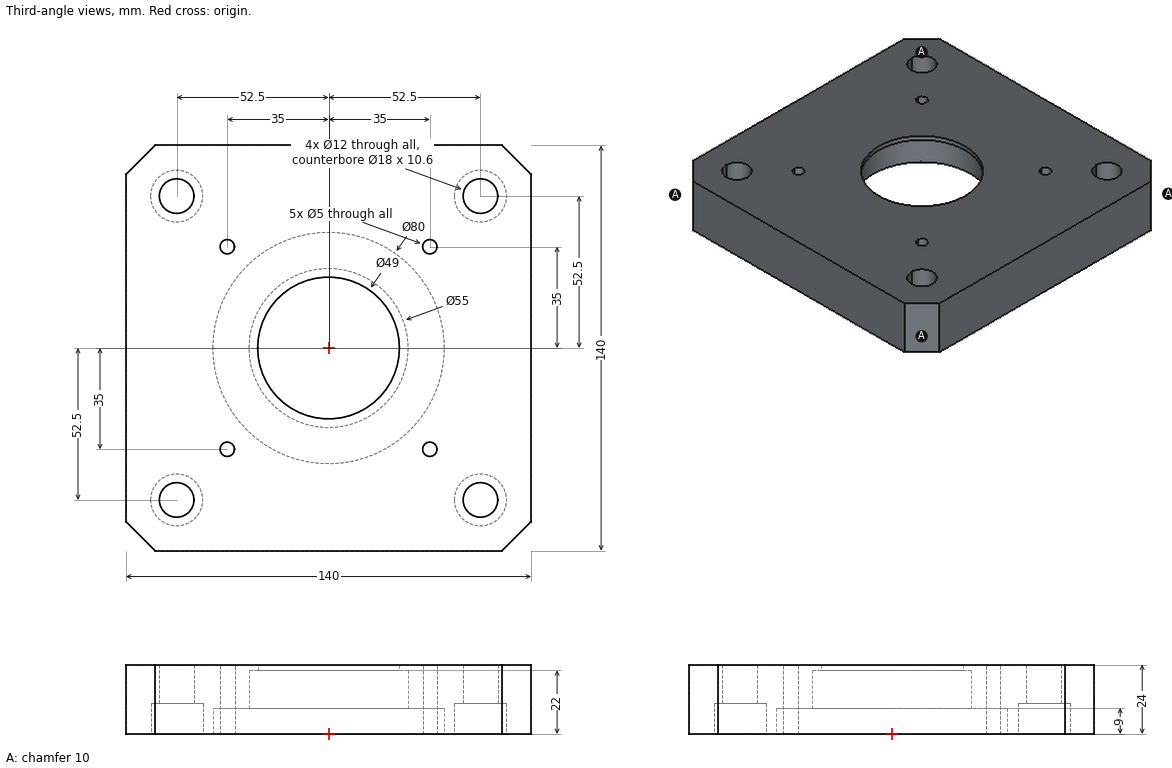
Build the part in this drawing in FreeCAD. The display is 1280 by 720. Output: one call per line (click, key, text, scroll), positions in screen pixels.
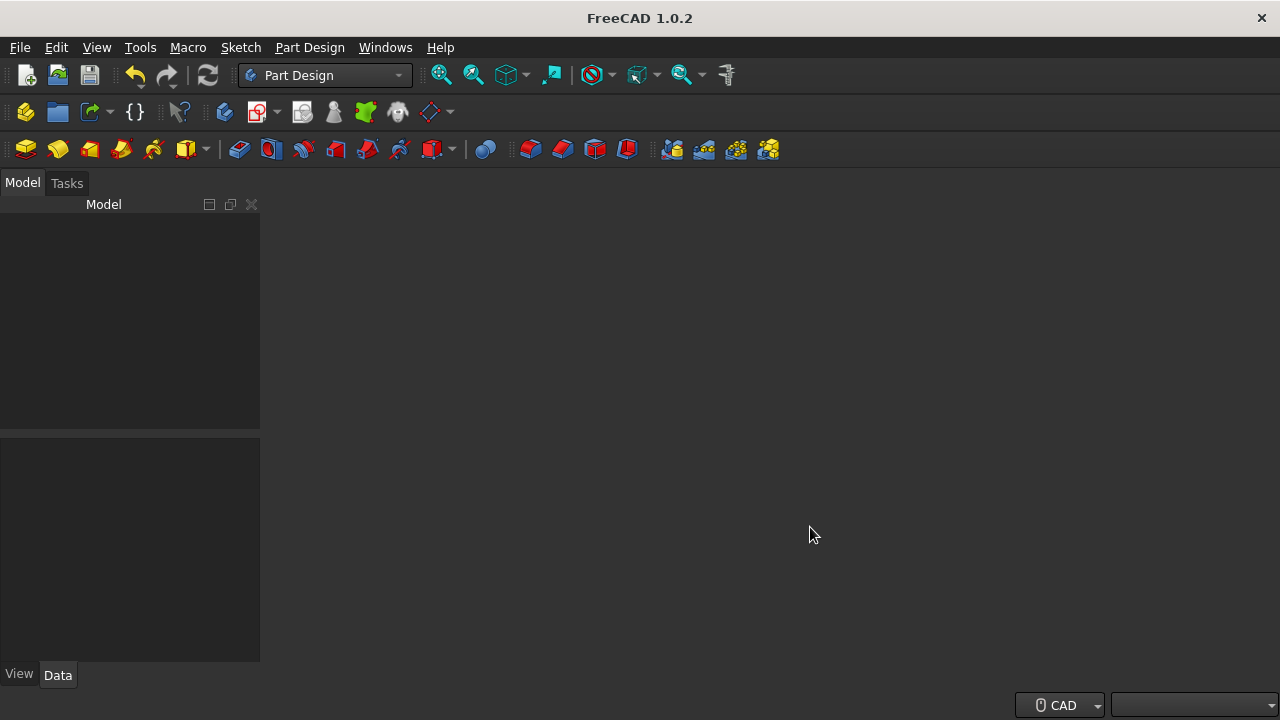
click(26, 76)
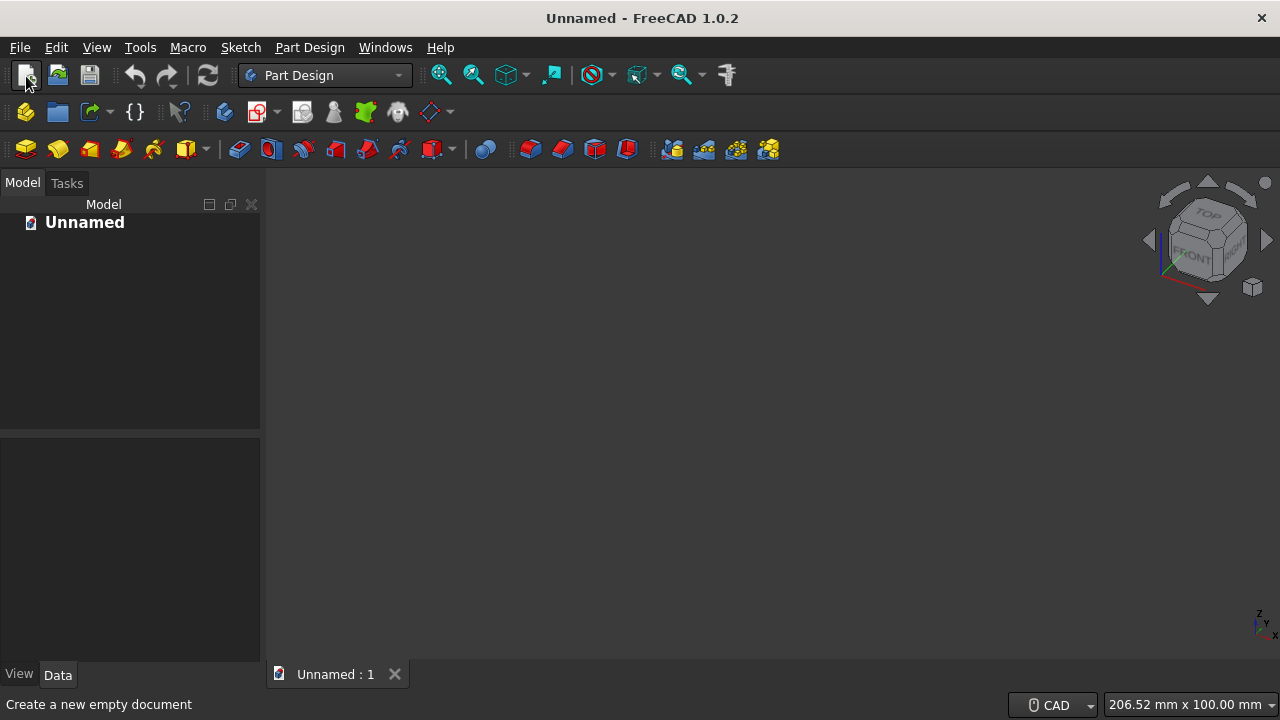
click(258, 112)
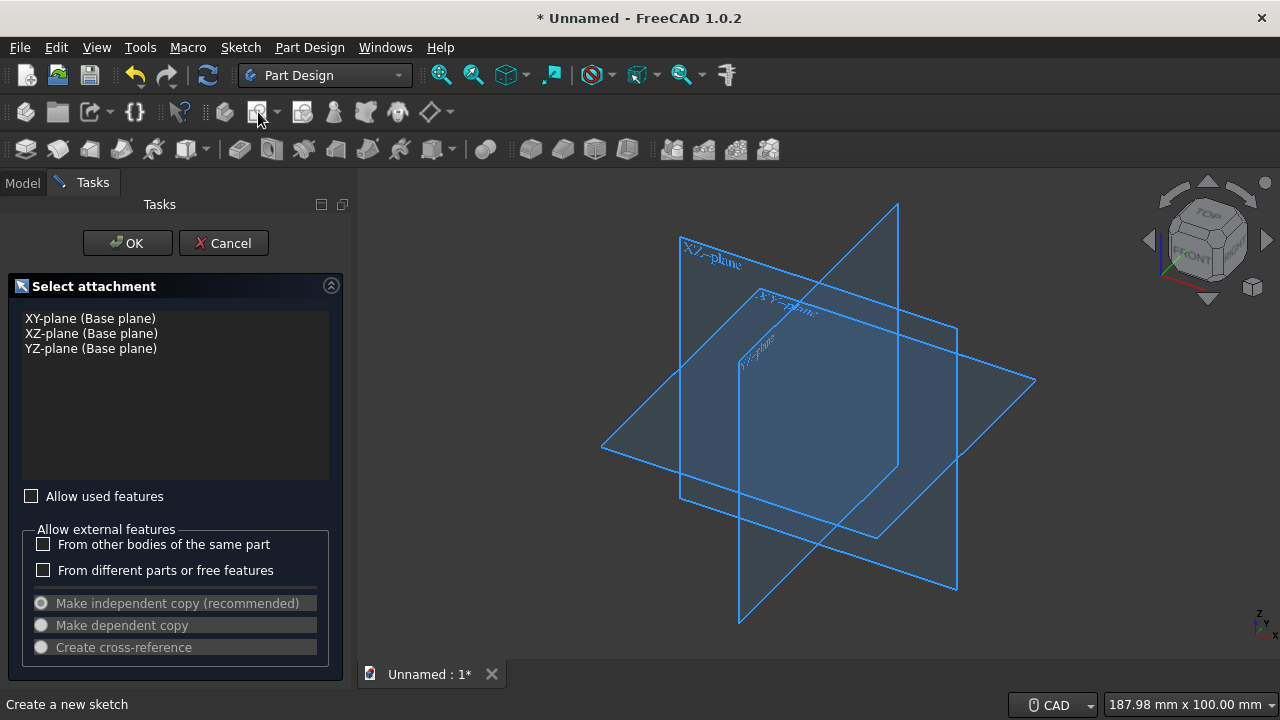
click(82, 318)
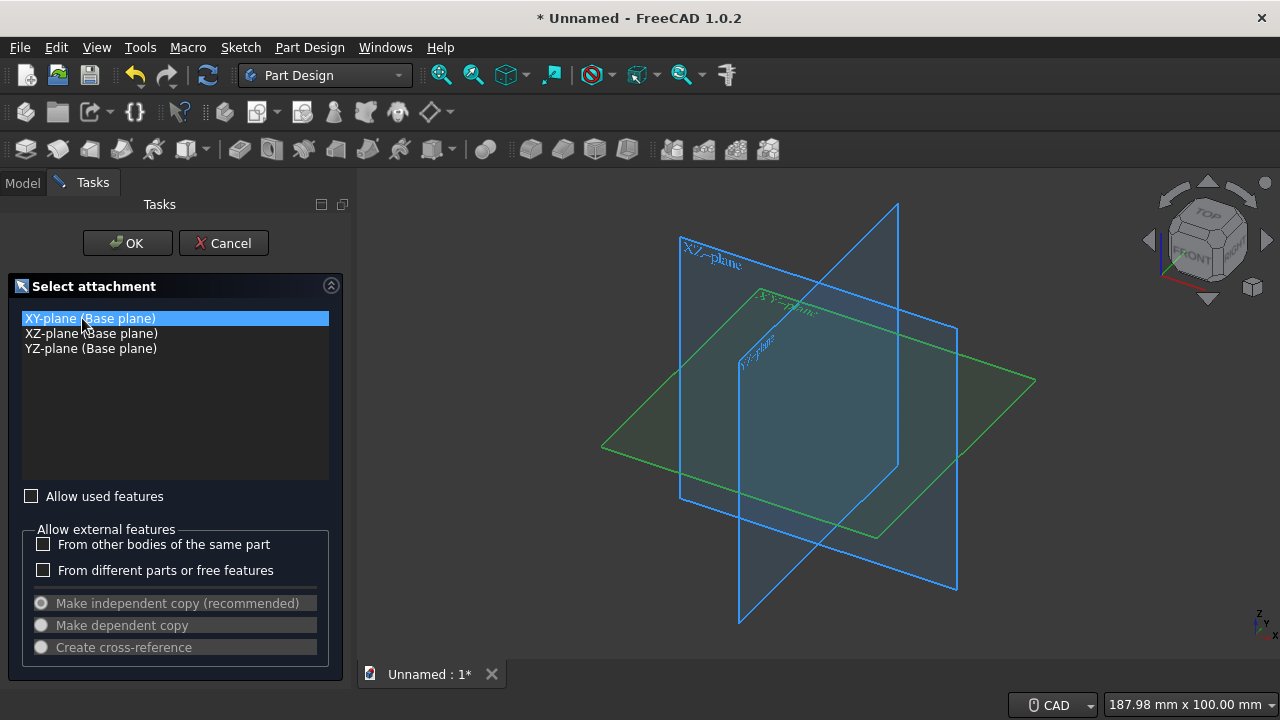
click(128, 243)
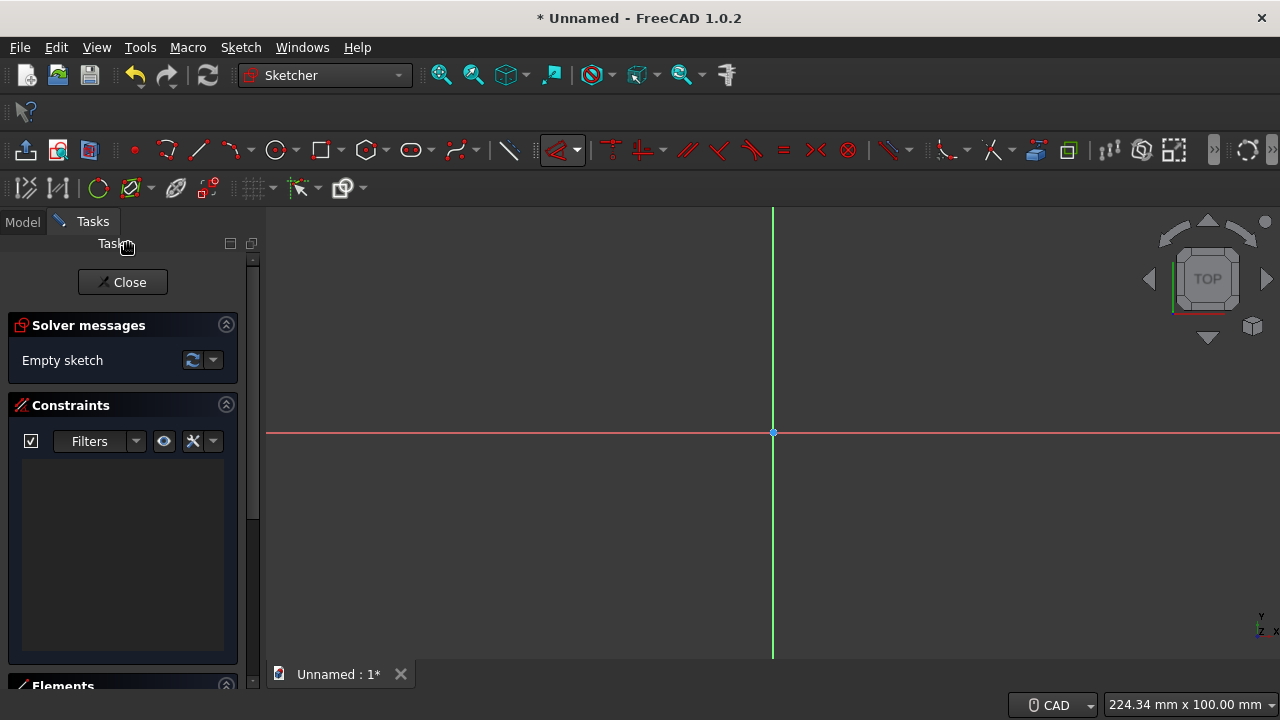
scroll(649, 433, down, 4)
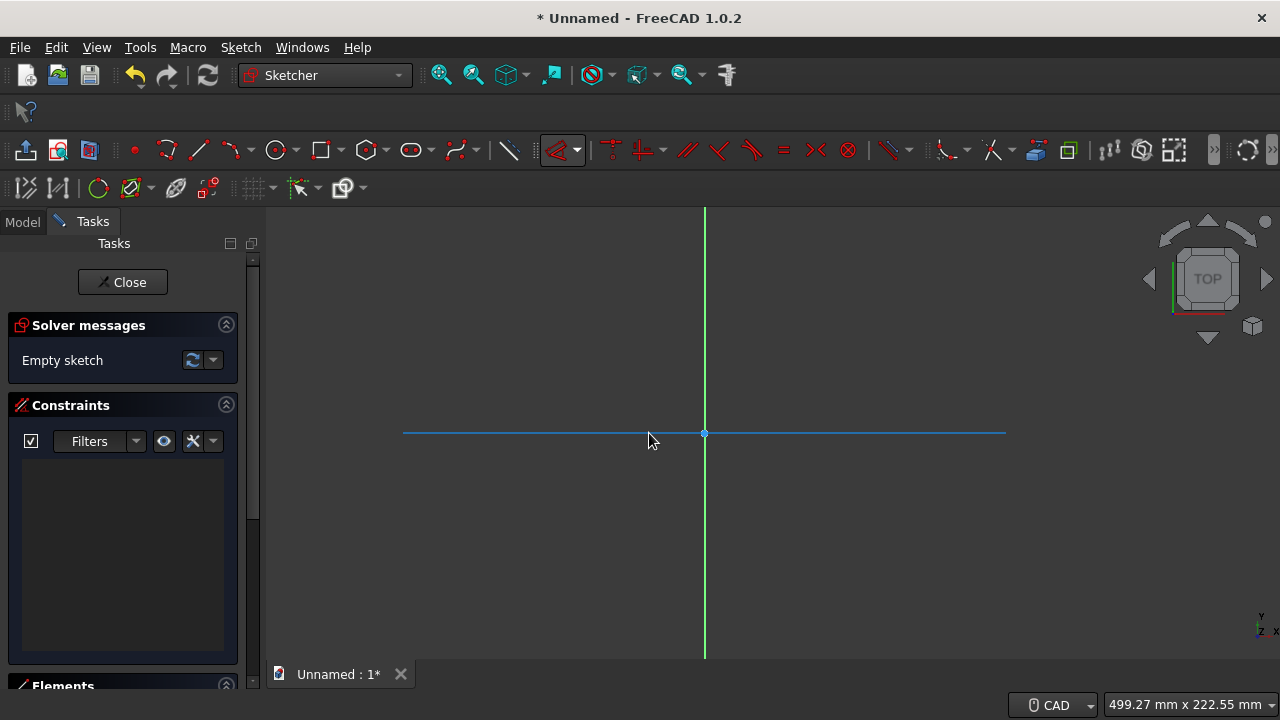
click(344, 150)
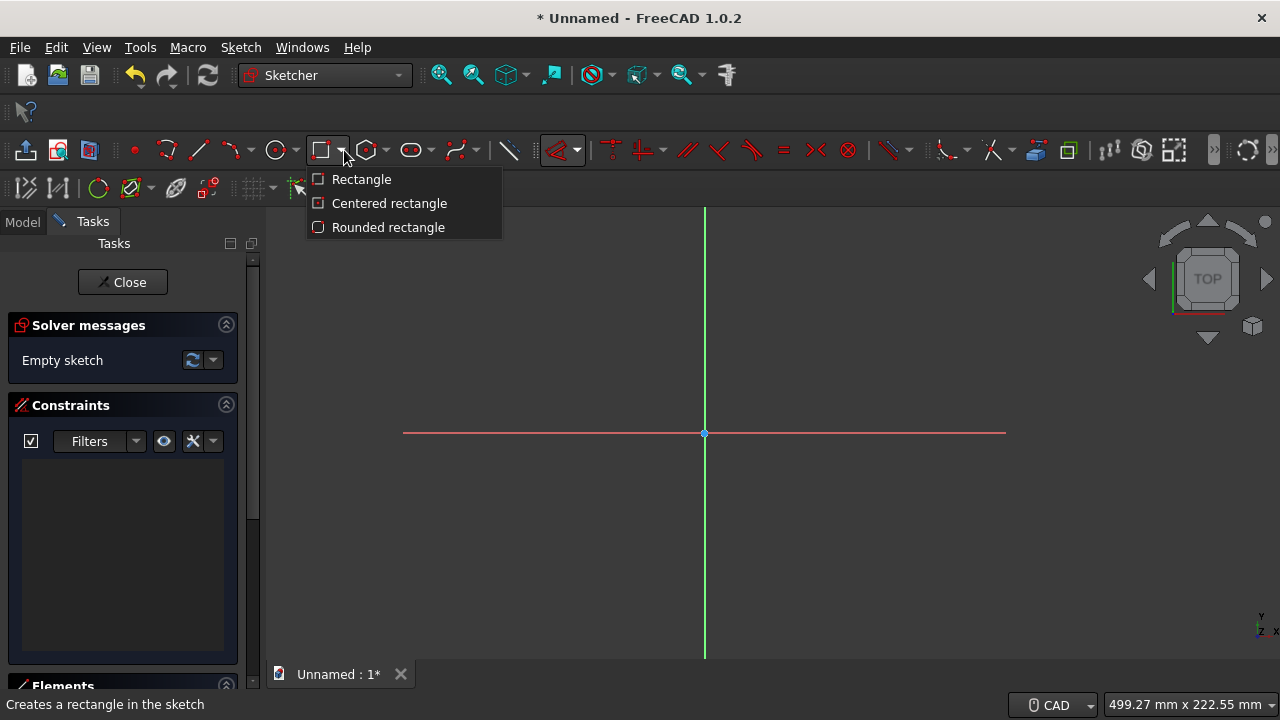
click(404, 203)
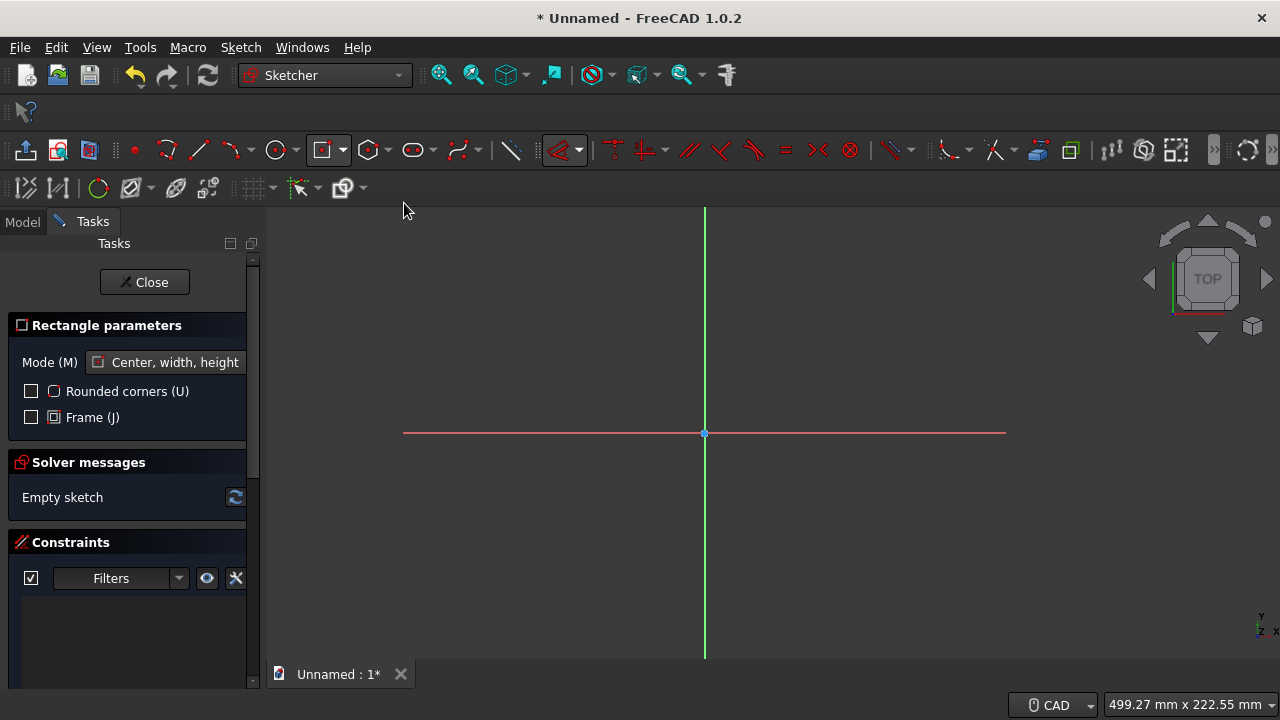
click(705, 433)
move(847, 291)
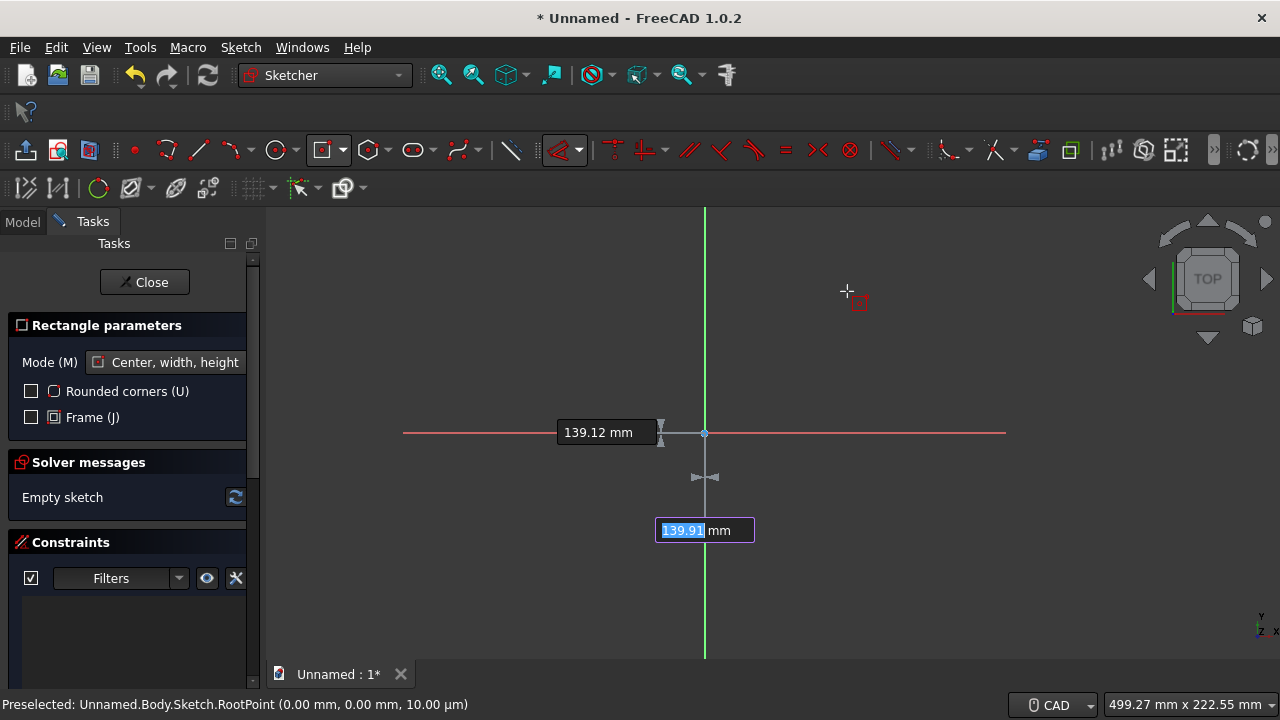
text(140)
key(Tab)
text(140)
key(Return)
key(Escape)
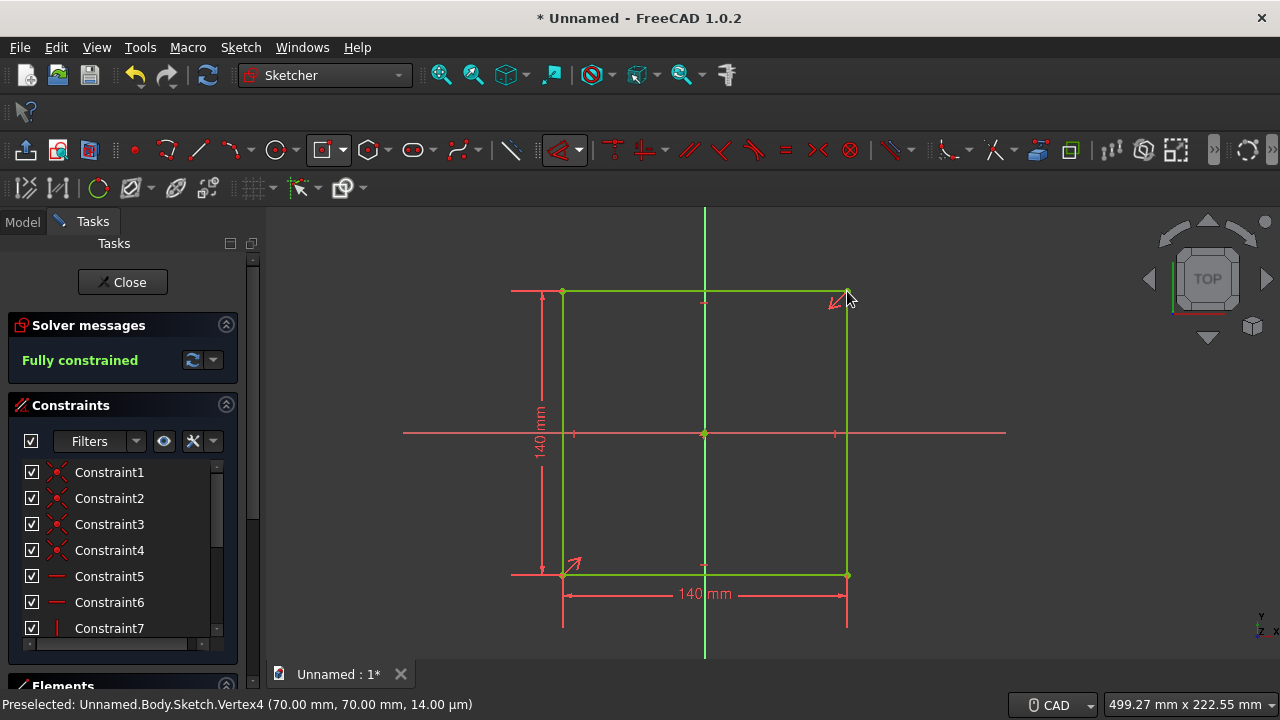
click(123, 282)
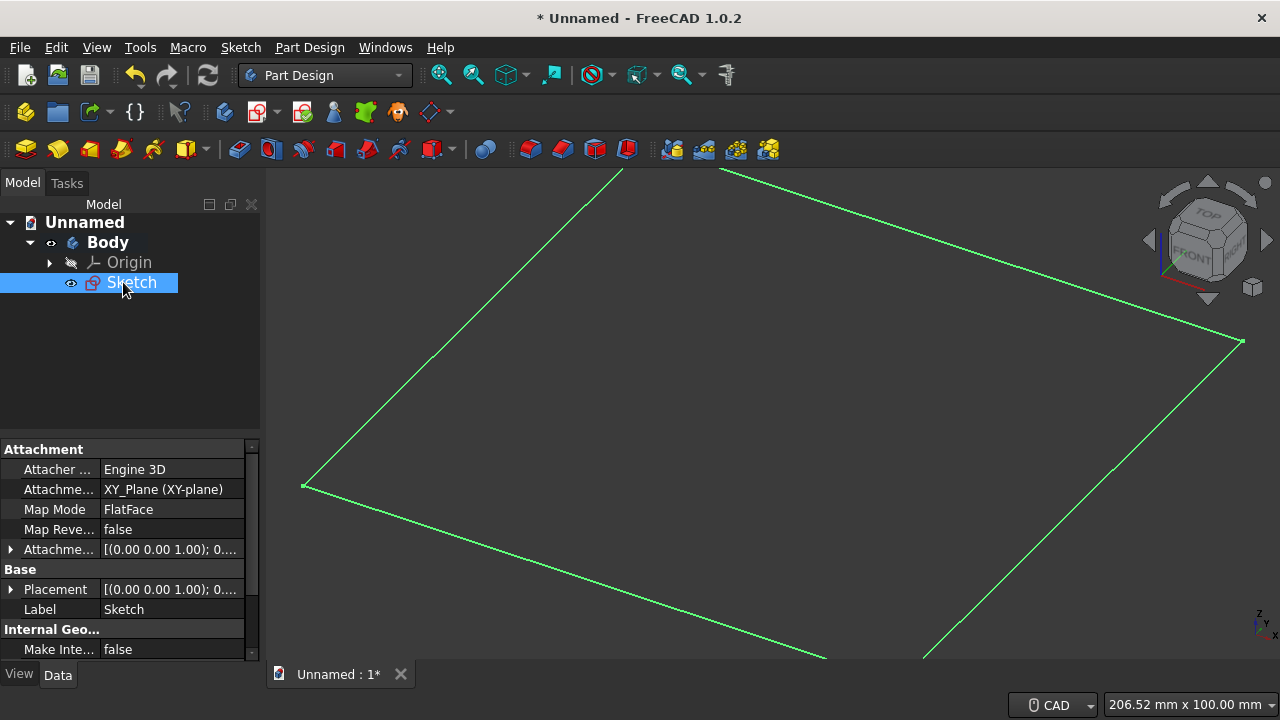
click(26, 150)